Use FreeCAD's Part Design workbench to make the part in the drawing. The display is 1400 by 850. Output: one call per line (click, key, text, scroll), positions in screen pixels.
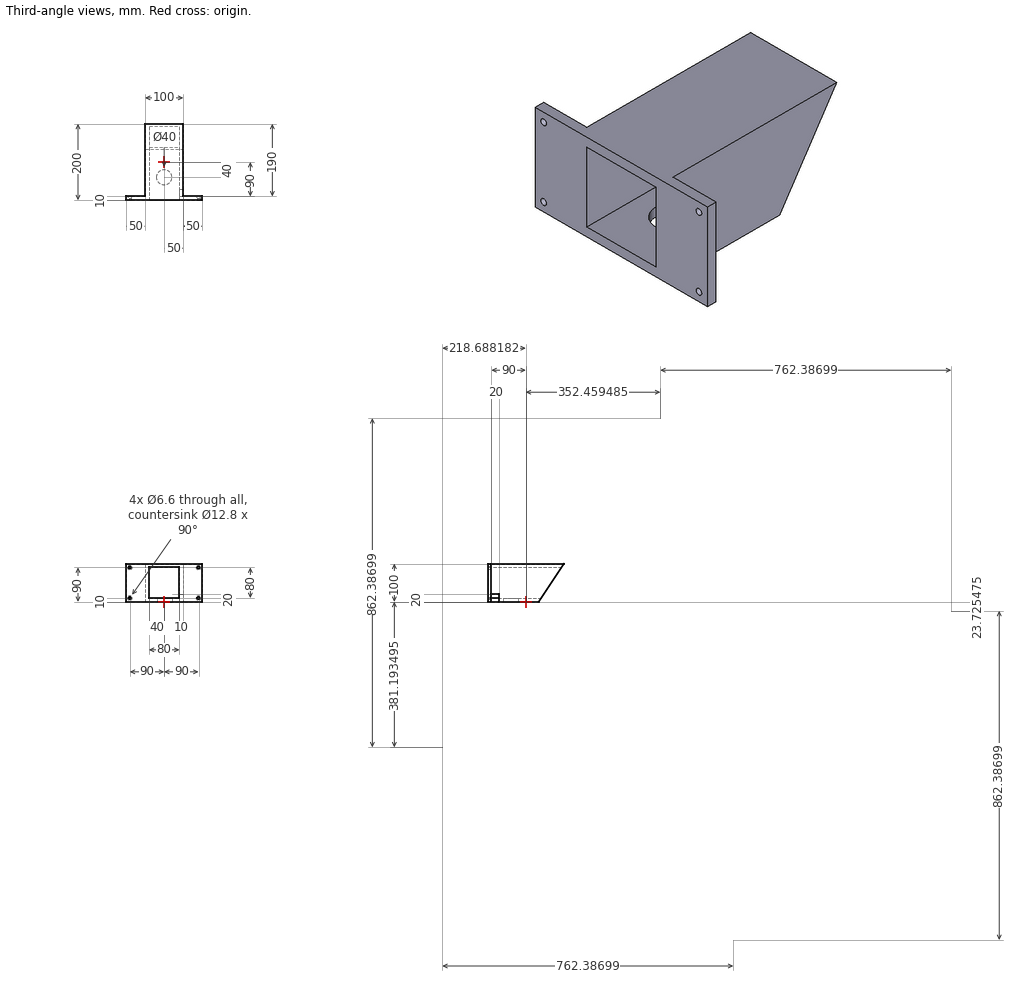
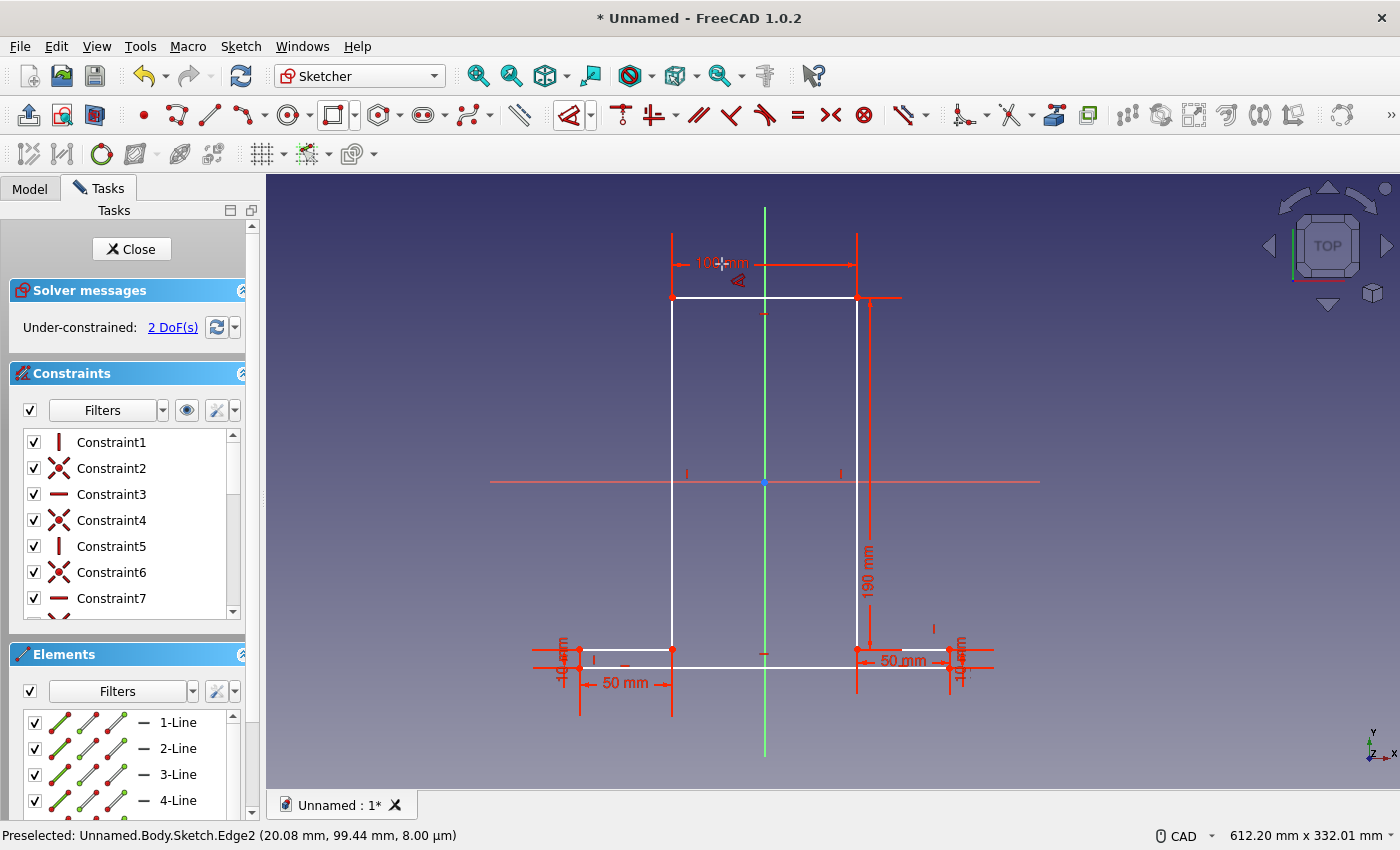
click(857, 650)
click(811, 684)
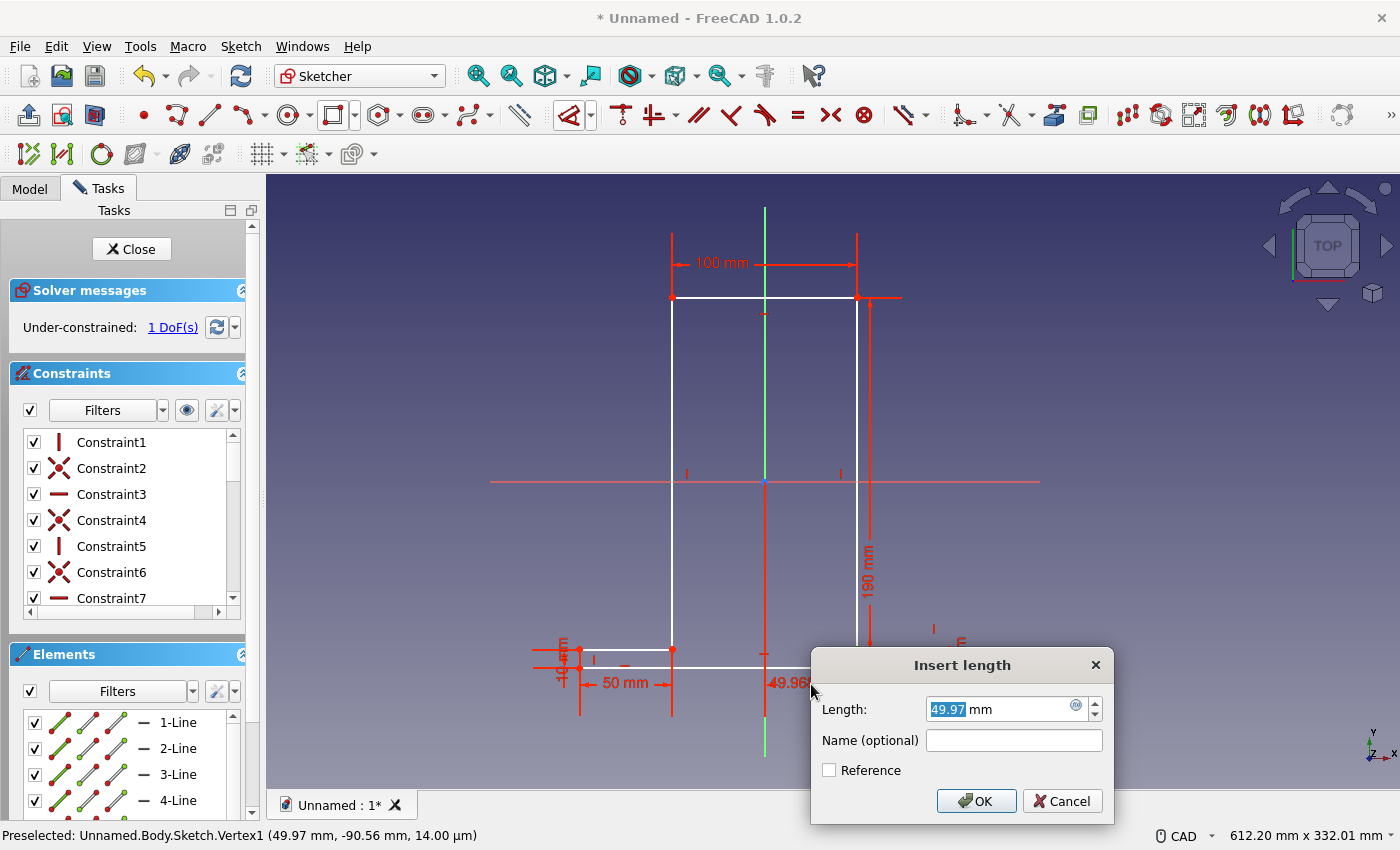
text(50)
key(Return)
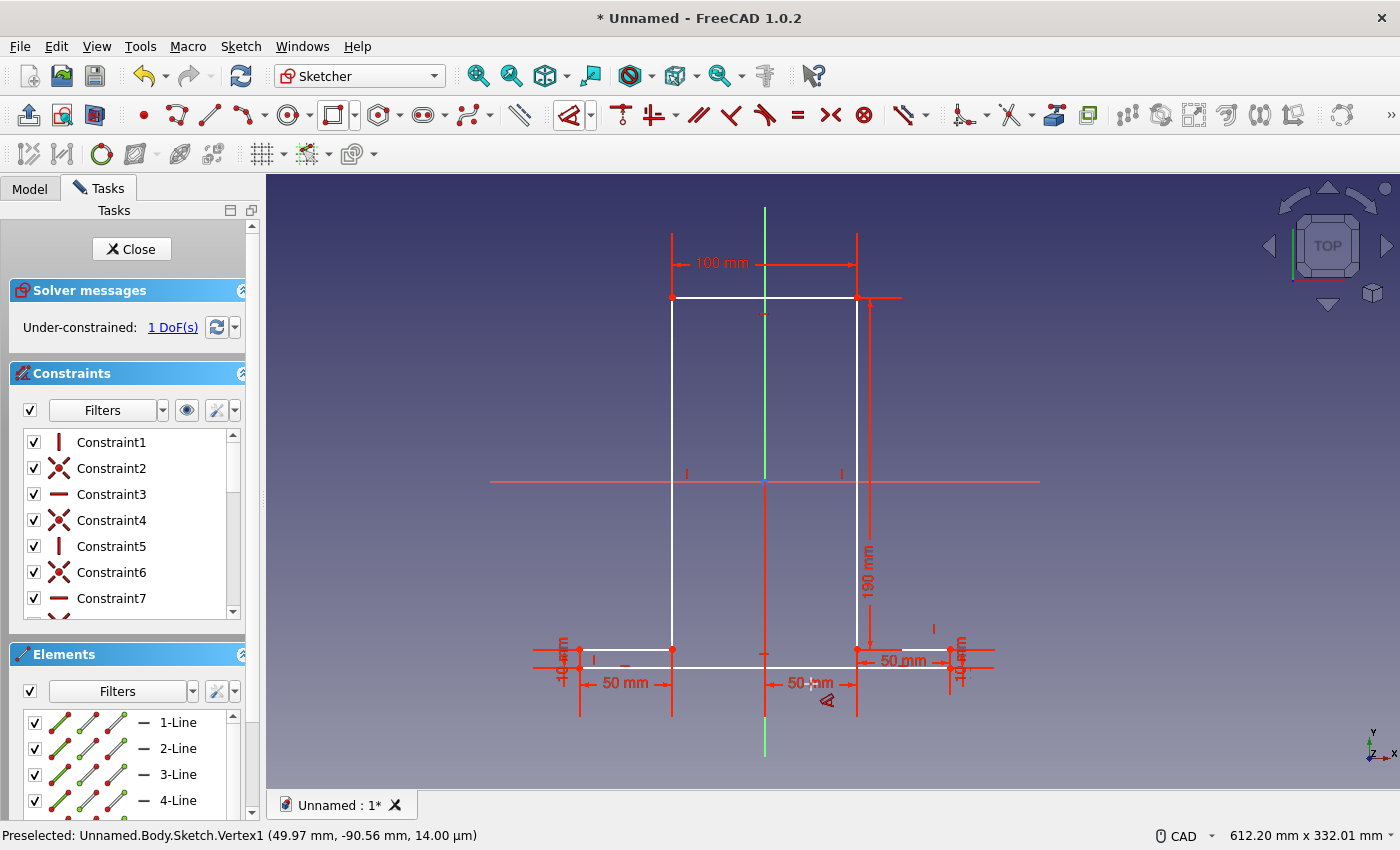
click(857, 650)
click(891, 527)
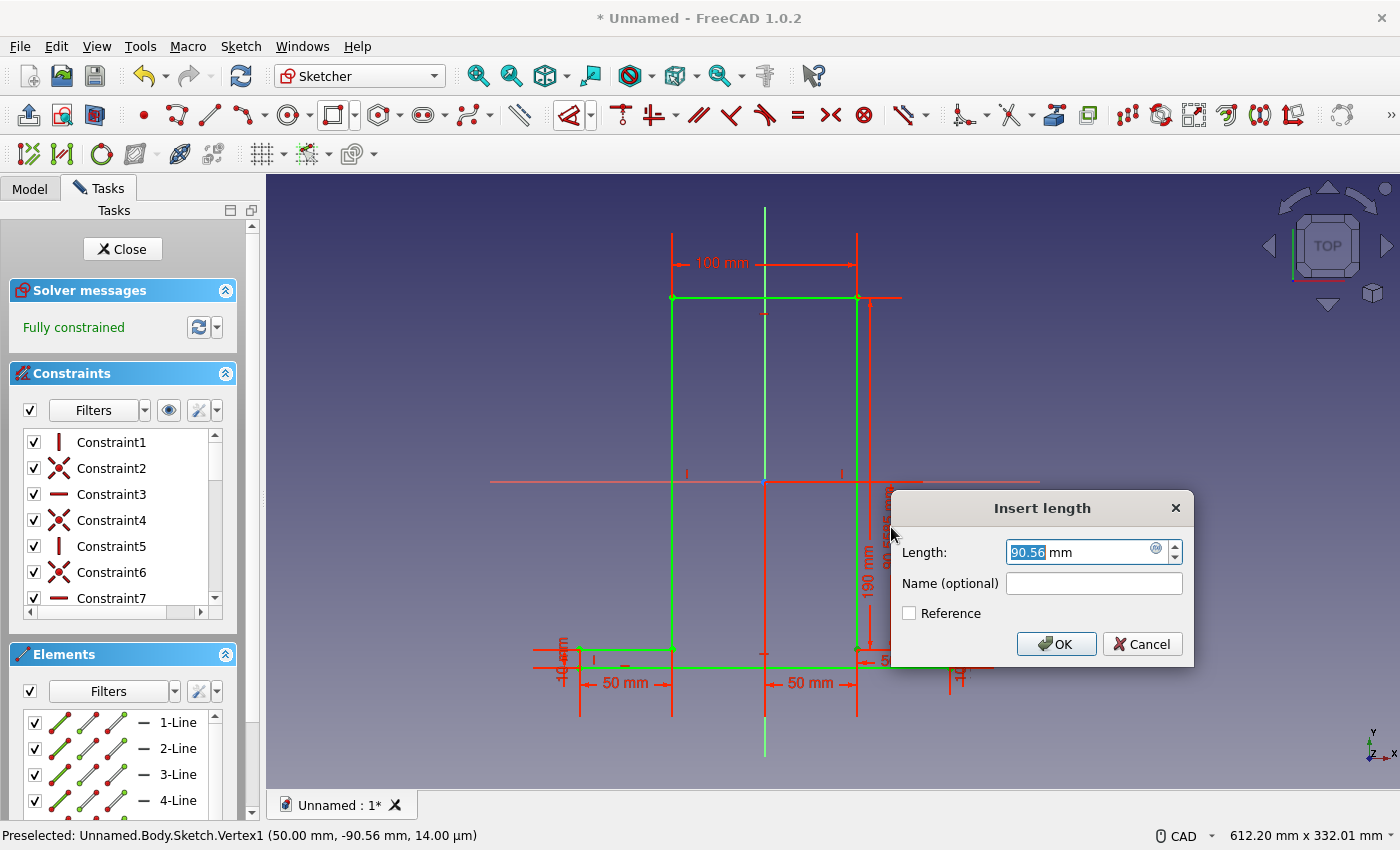
text(90)
key(Return)
key(Escape)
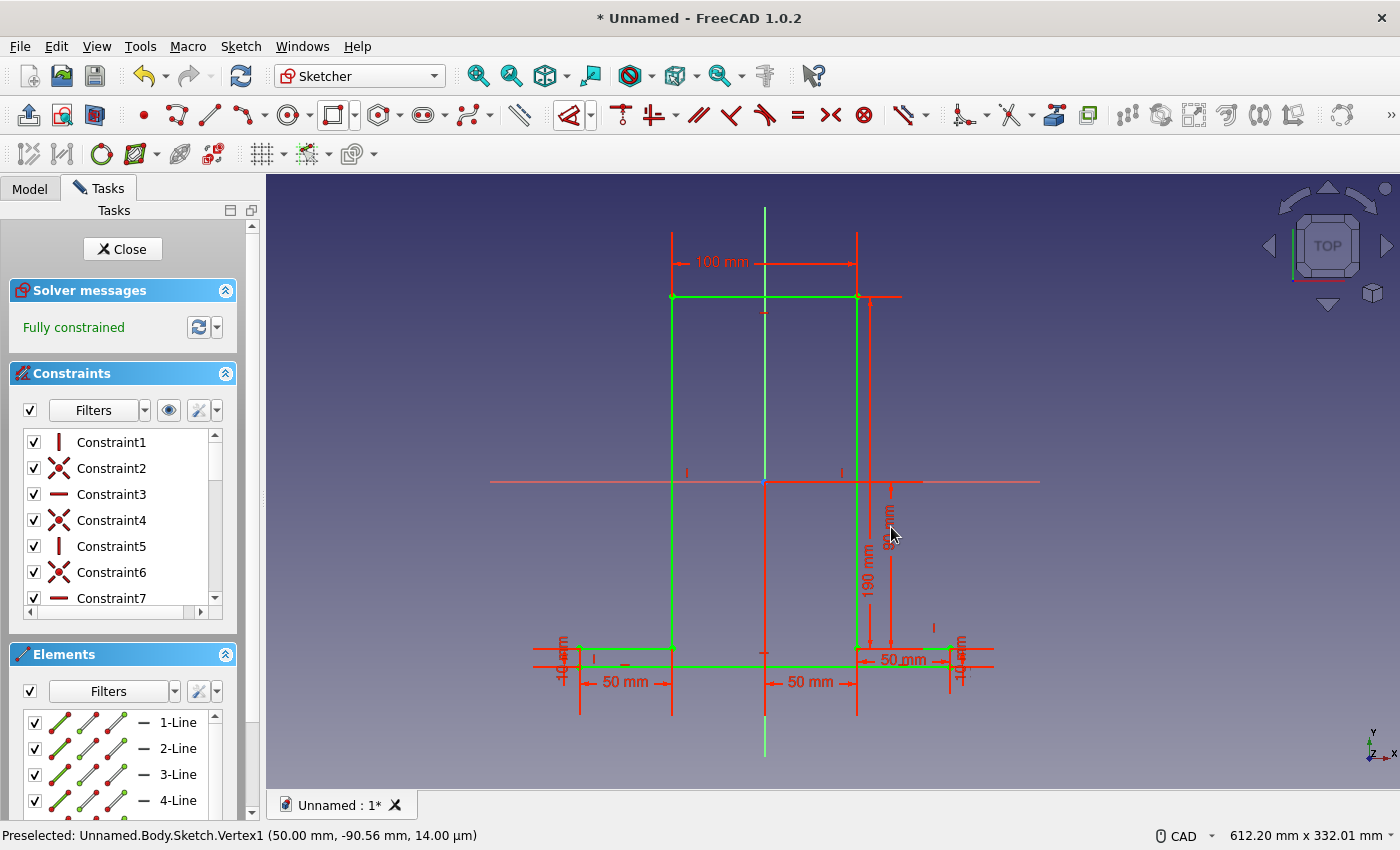
click(123, 249)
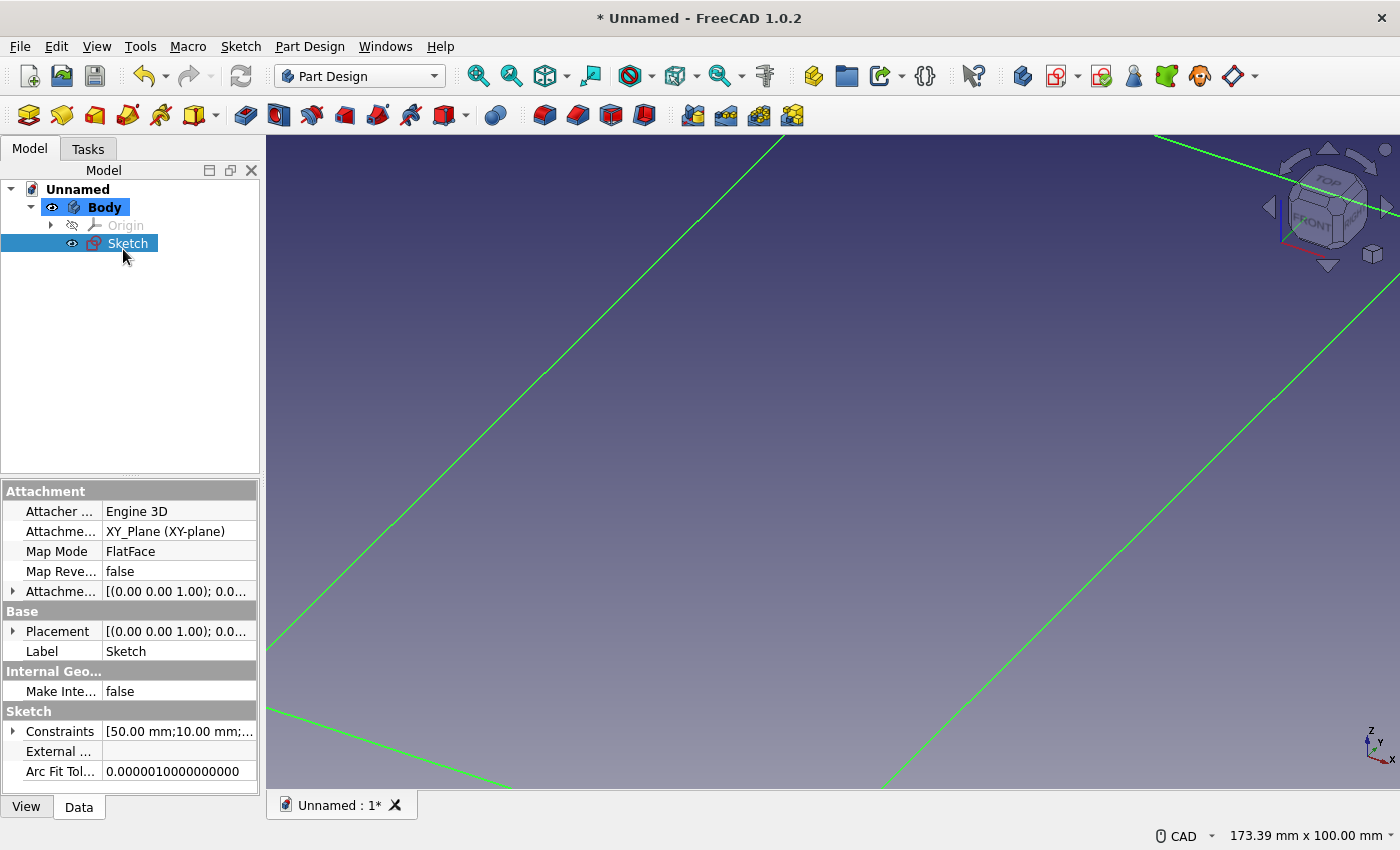
click(29, 116)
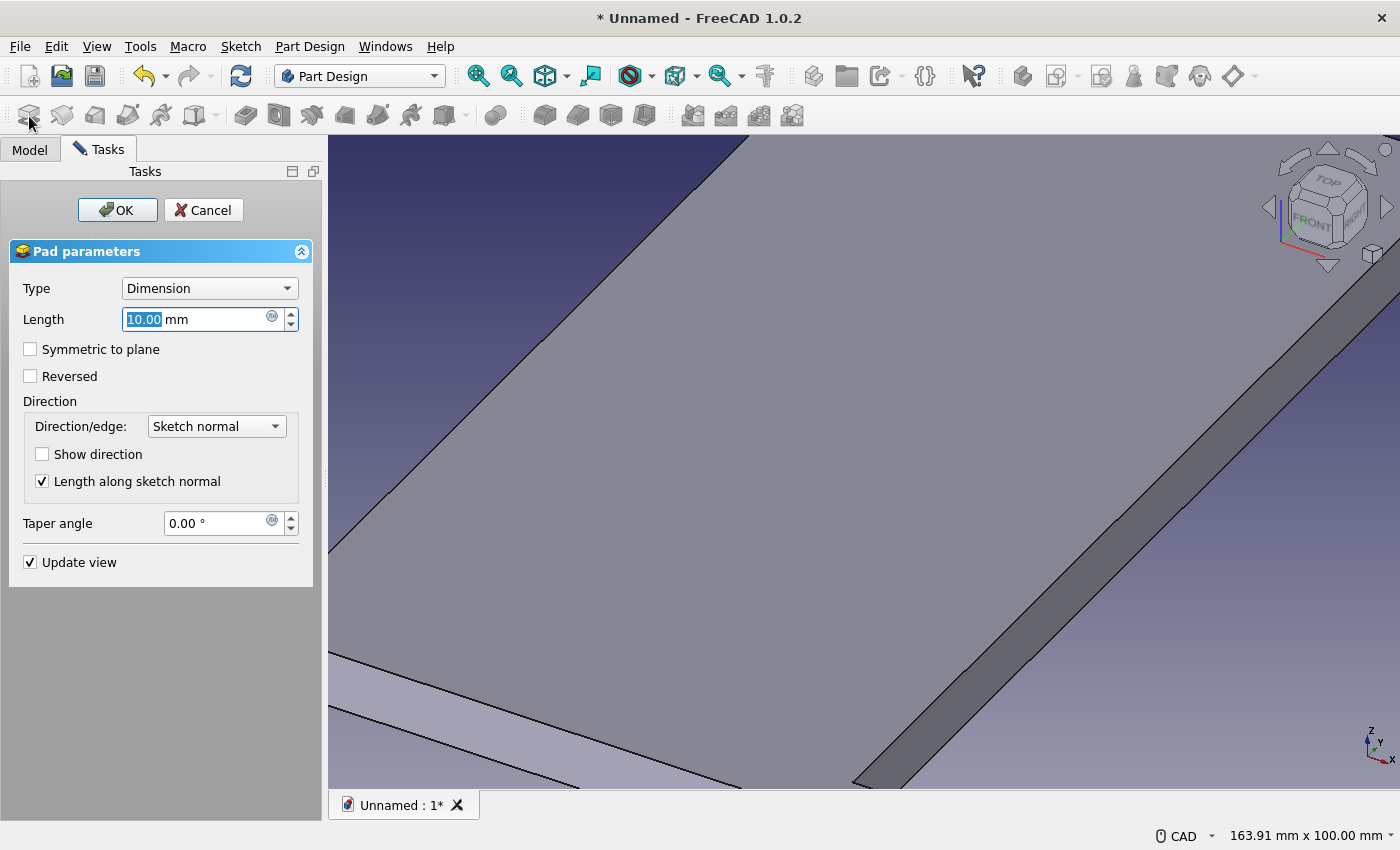
text(100)
key(Tab)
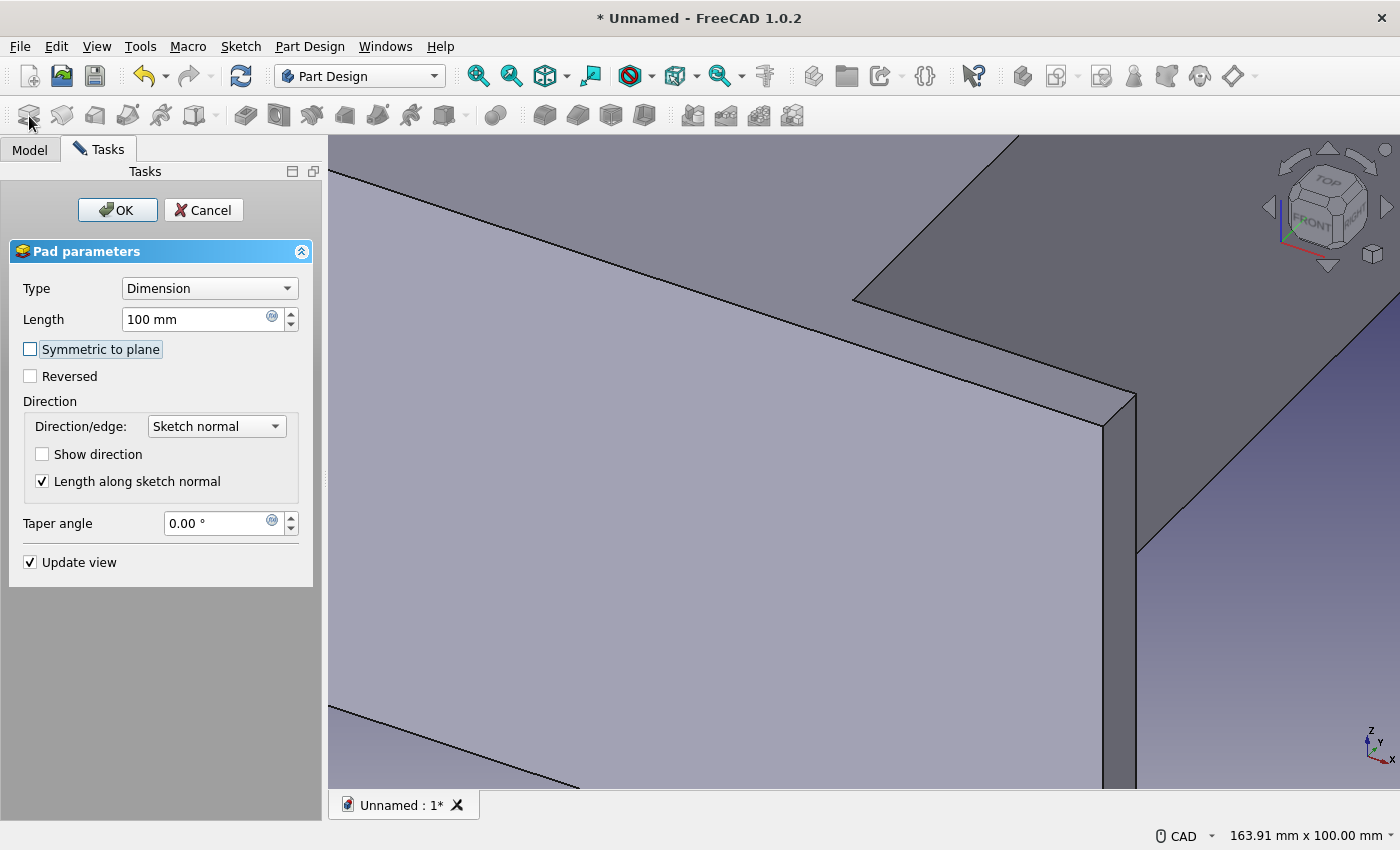
click(118, 210)